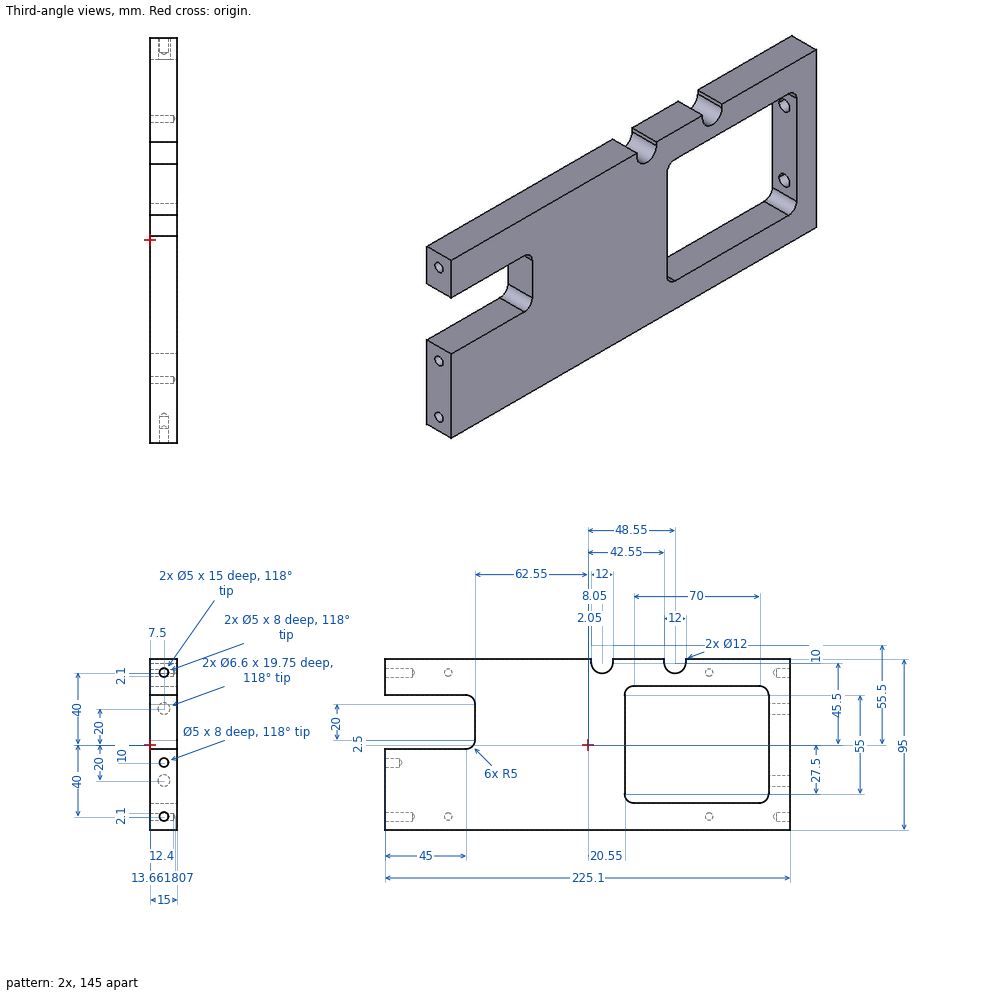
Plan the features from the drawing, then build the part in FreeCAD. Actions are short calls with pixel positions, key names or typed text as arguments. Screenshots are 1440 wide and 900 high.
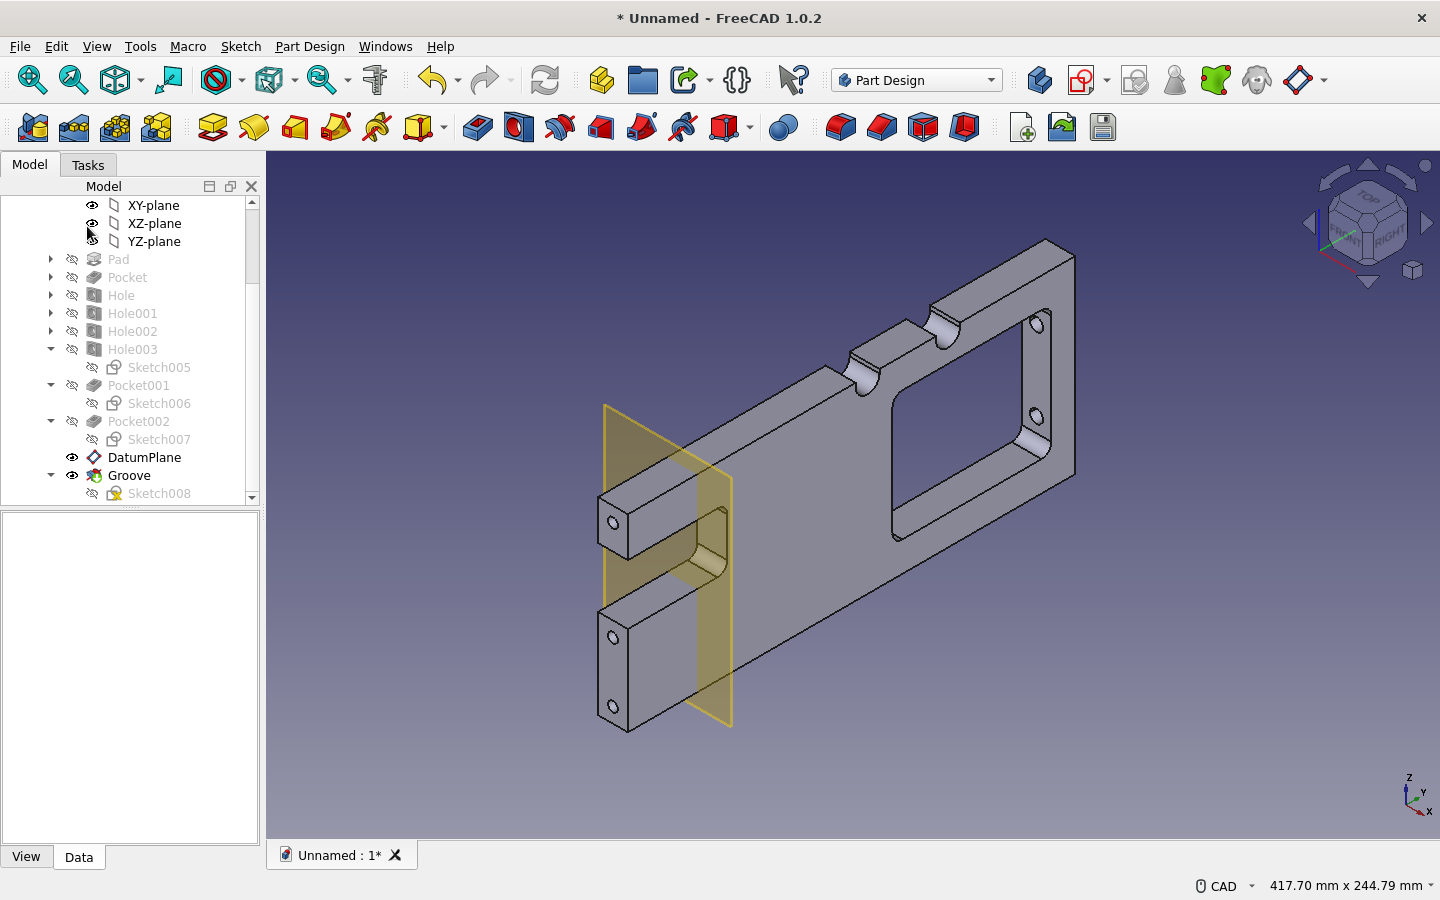
click(117, 457)
key(space)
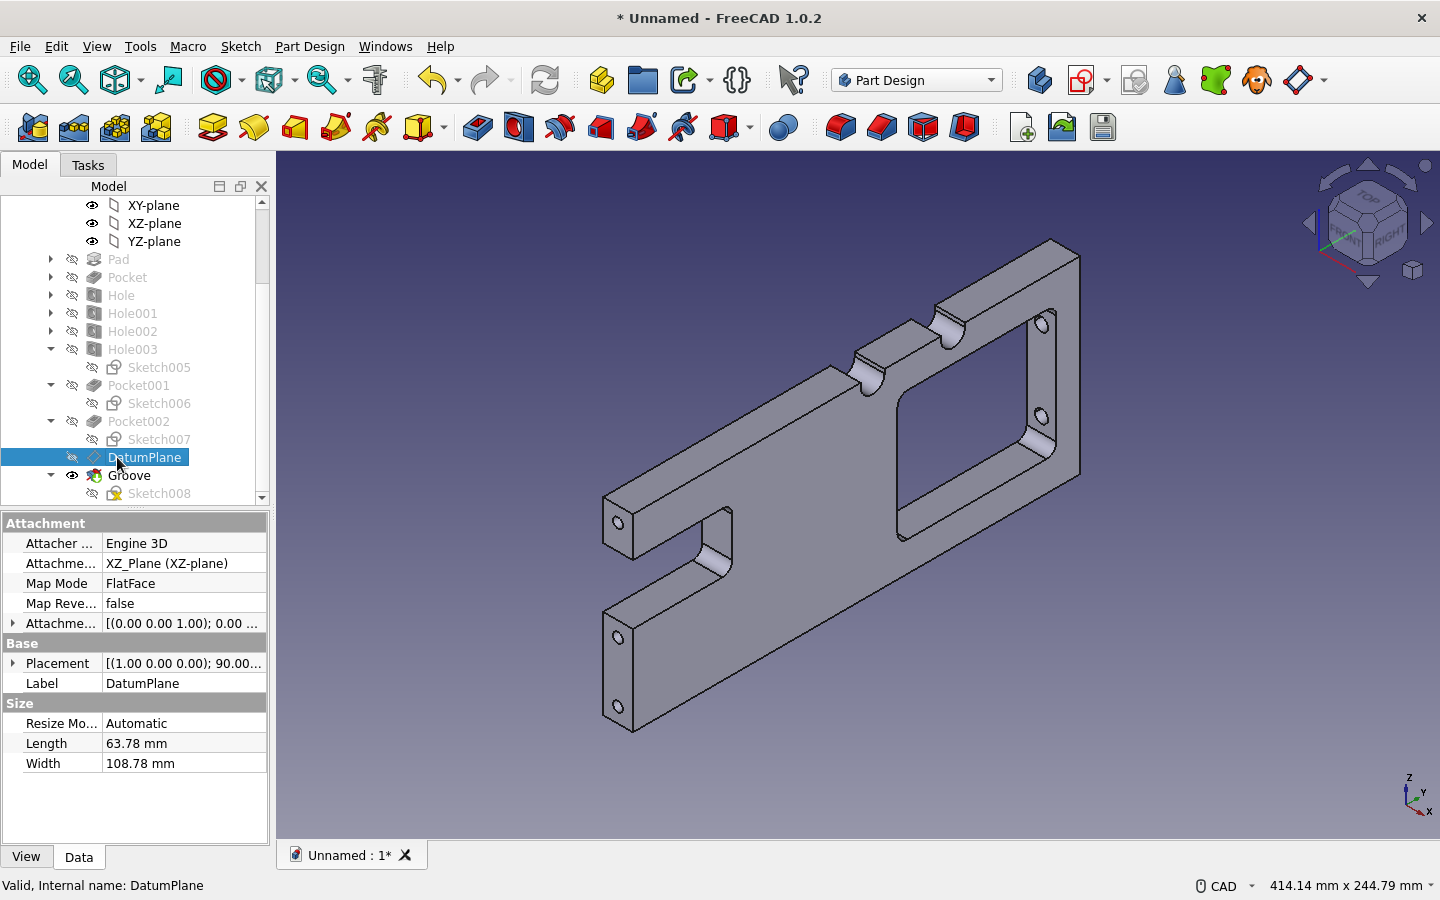
click(117, 475)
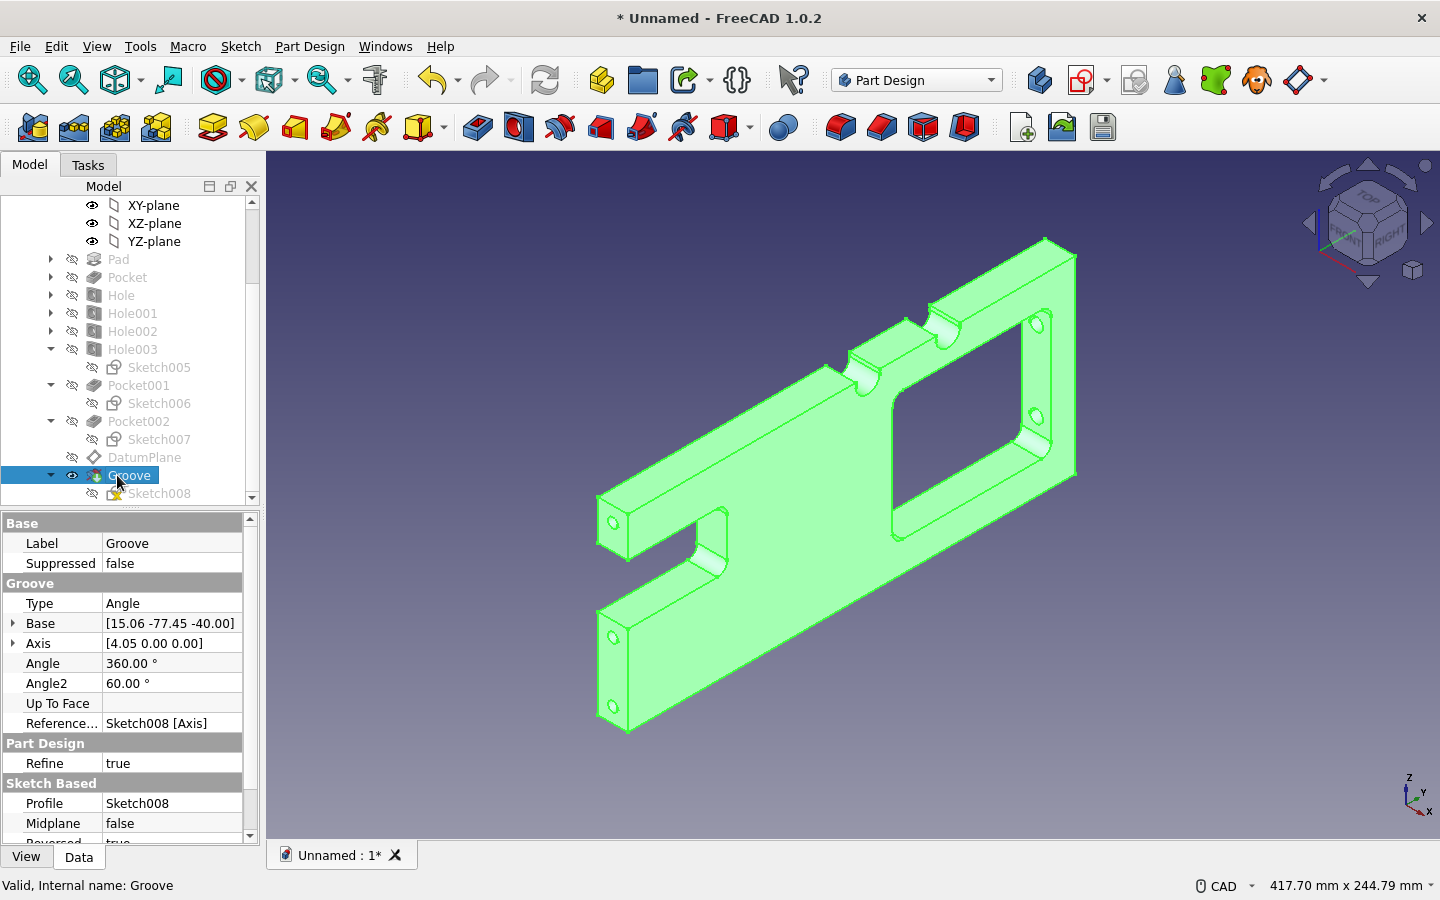
click(74, 128)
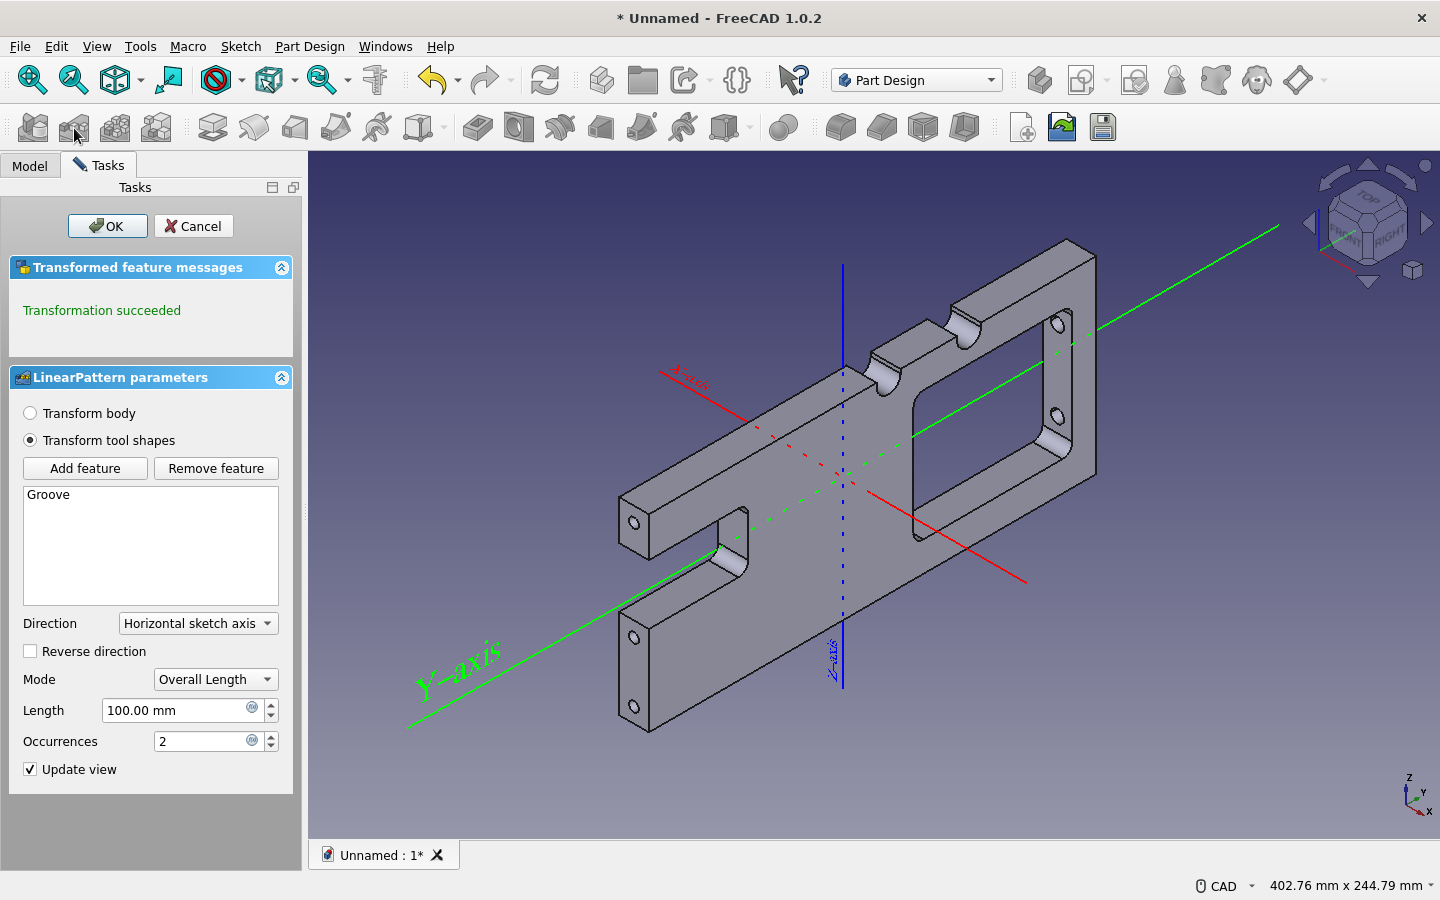
click(199, 624)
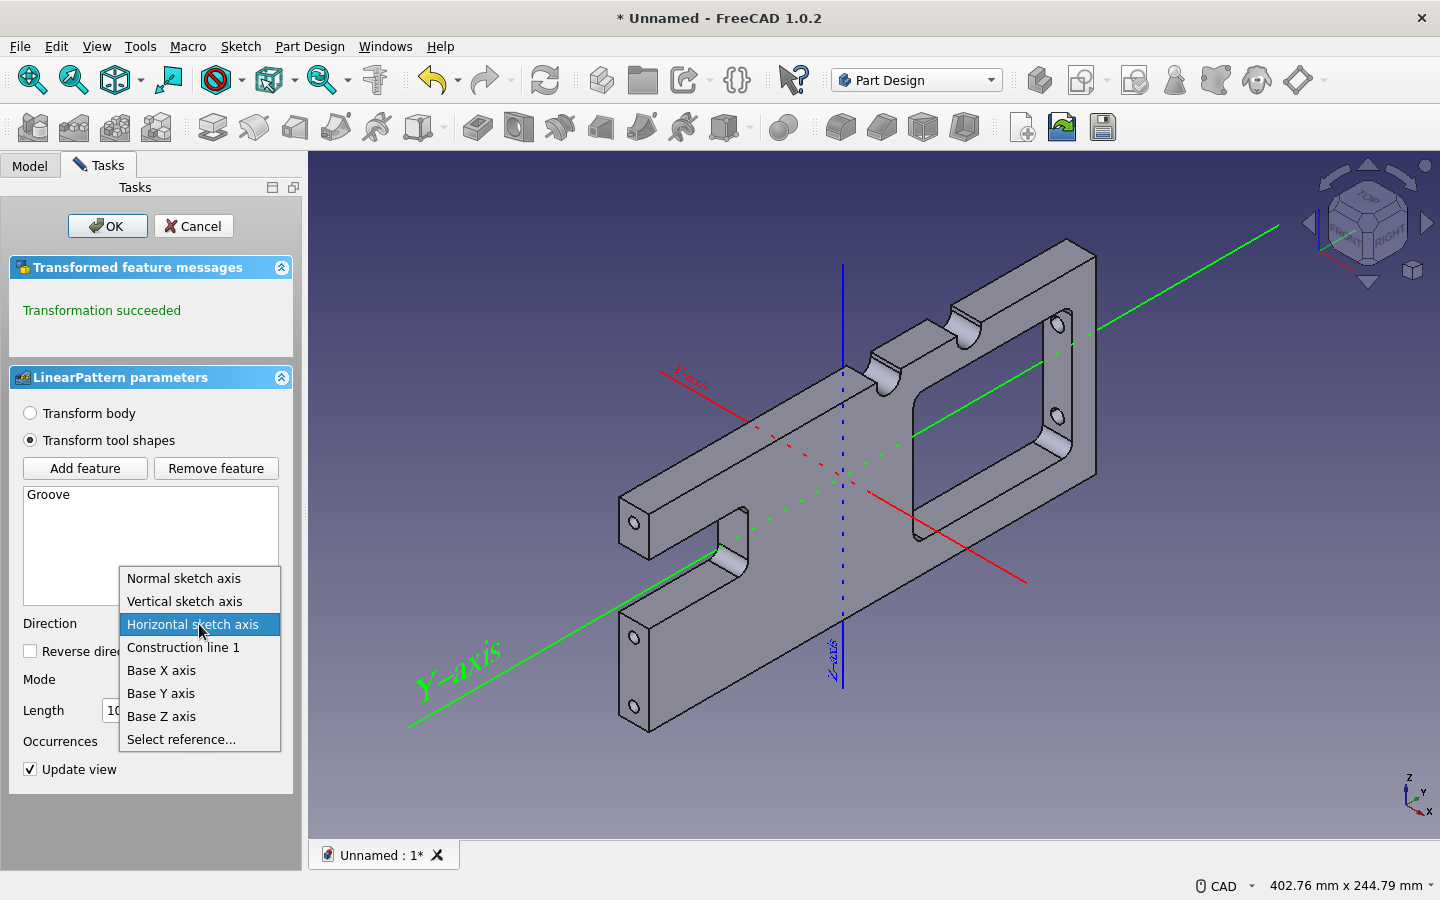
click(198, 694)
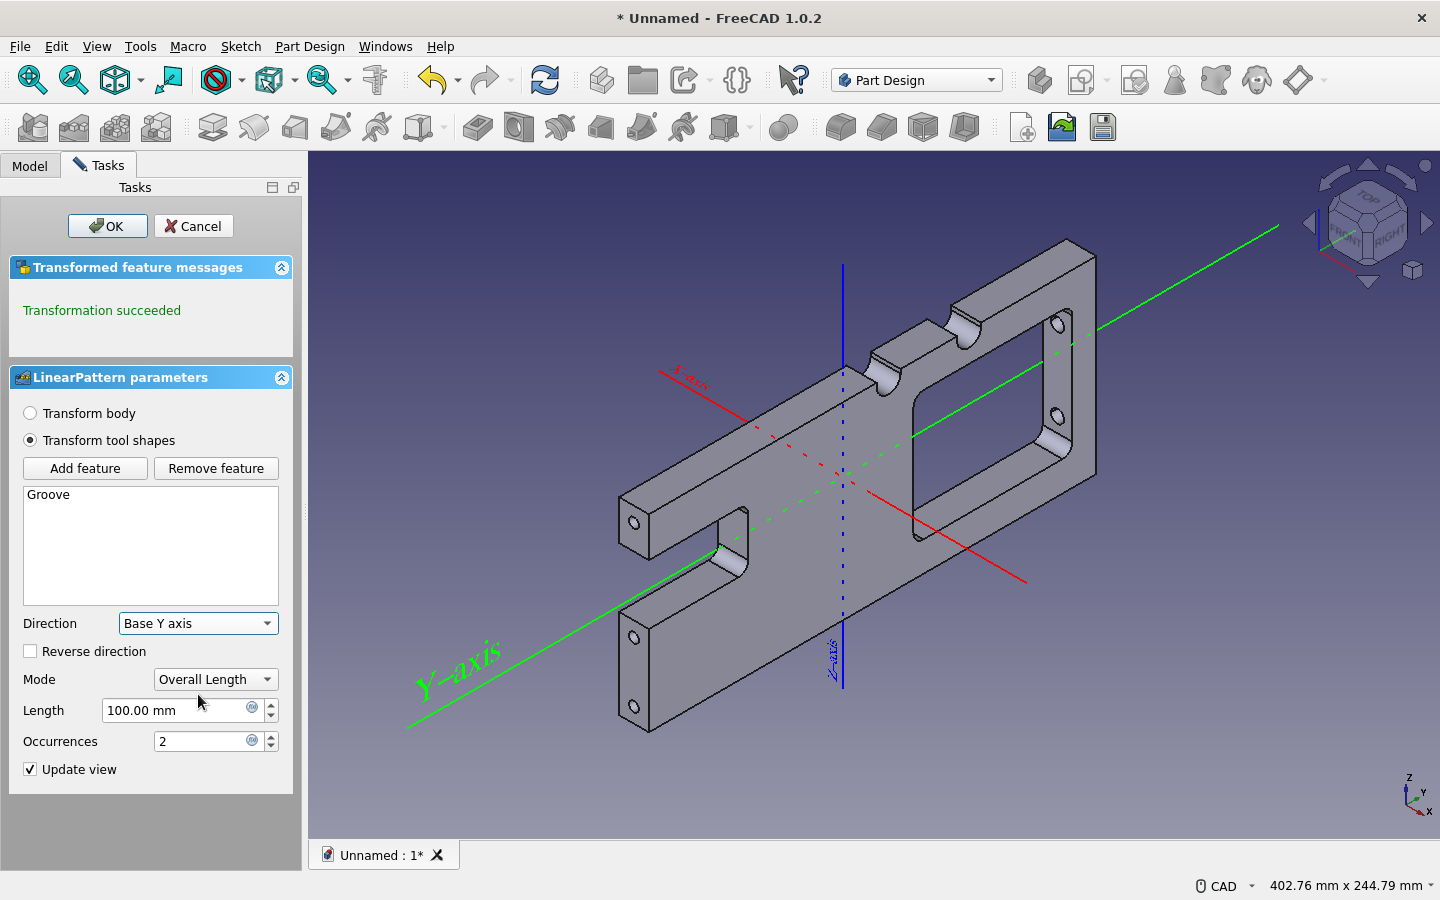
click(216, 680)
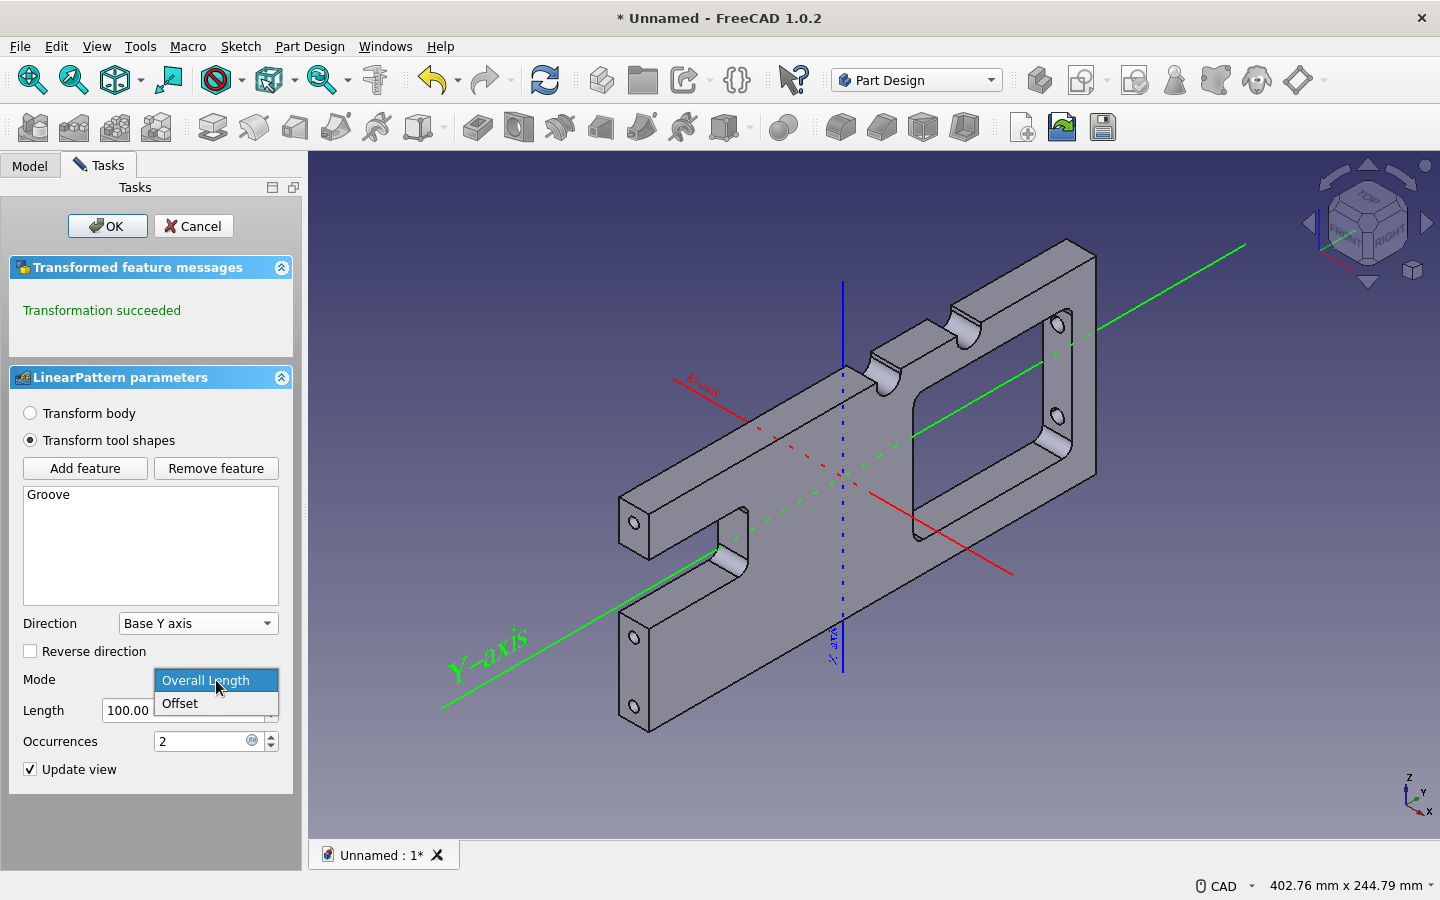
click(214, 704)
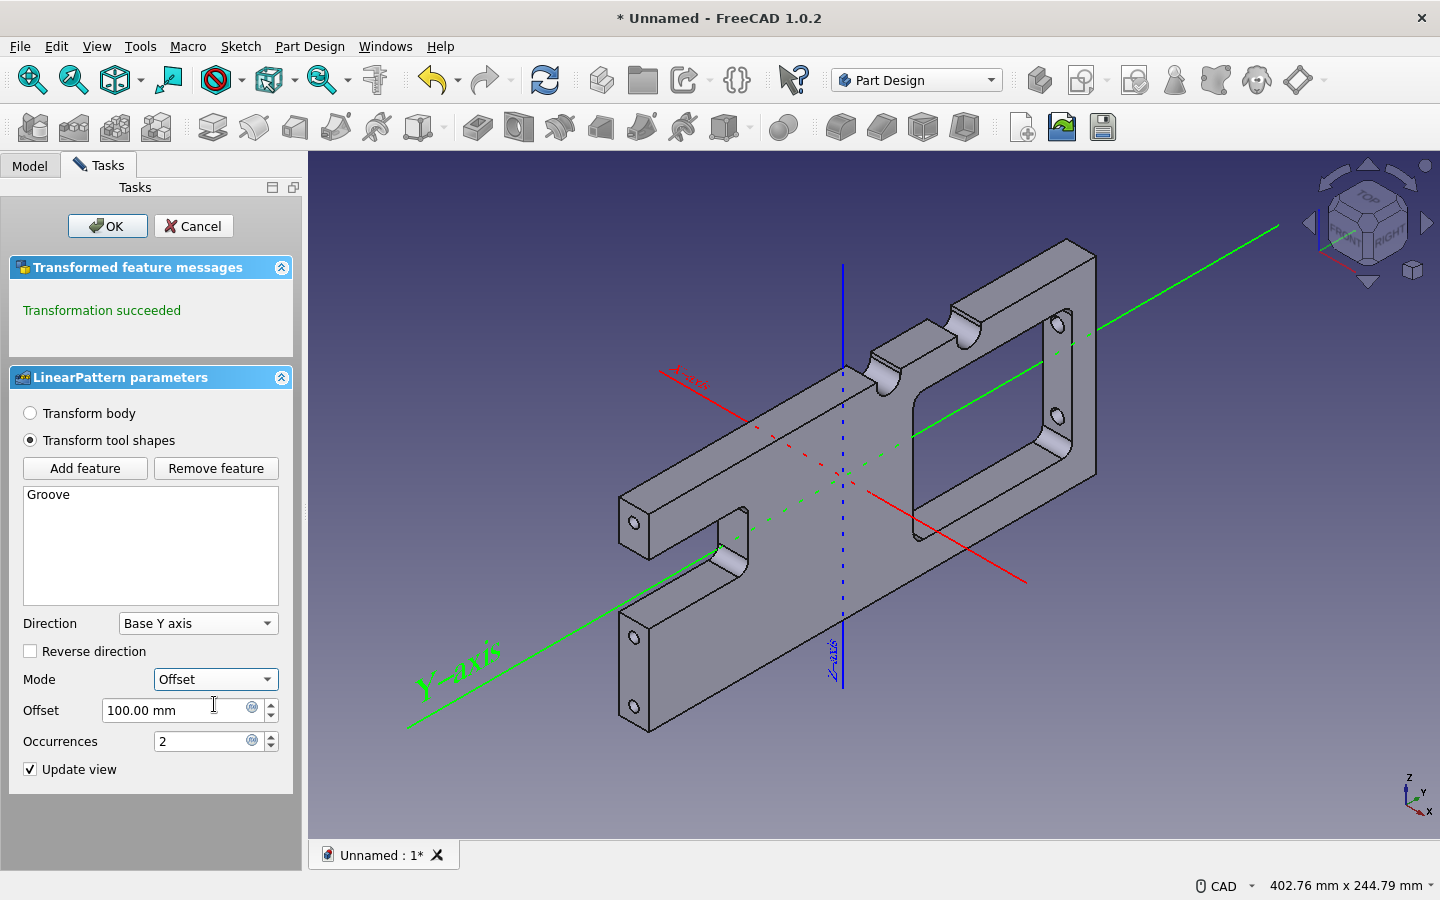
triple_click(184, 710)